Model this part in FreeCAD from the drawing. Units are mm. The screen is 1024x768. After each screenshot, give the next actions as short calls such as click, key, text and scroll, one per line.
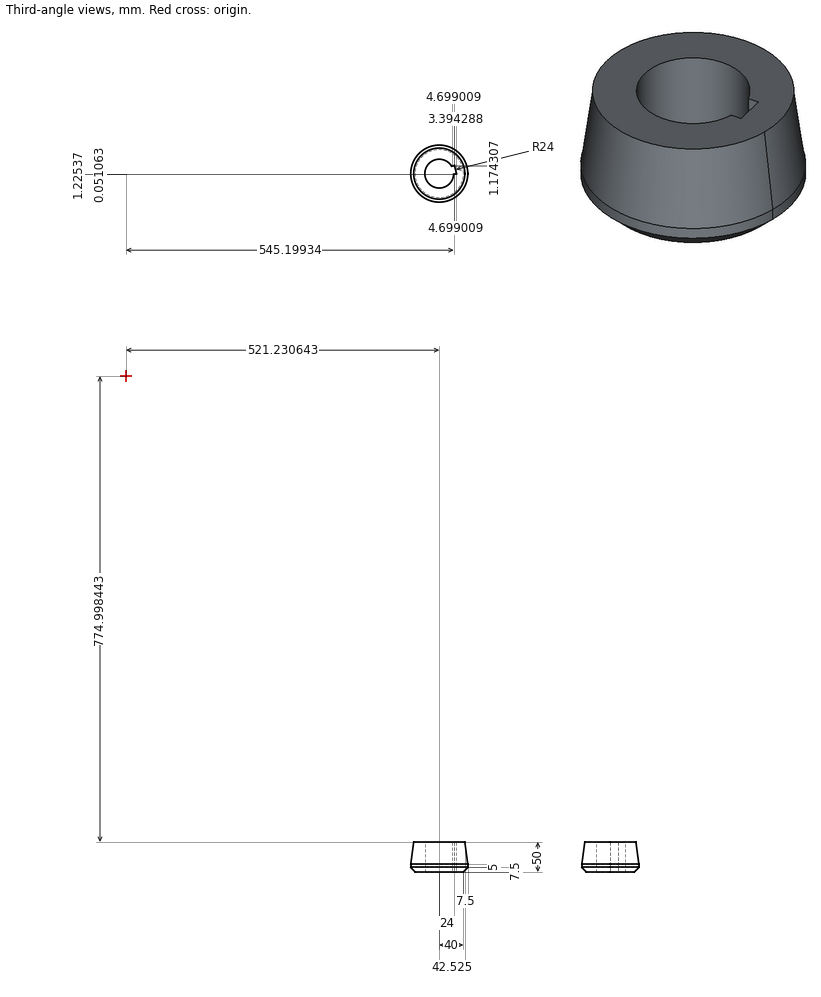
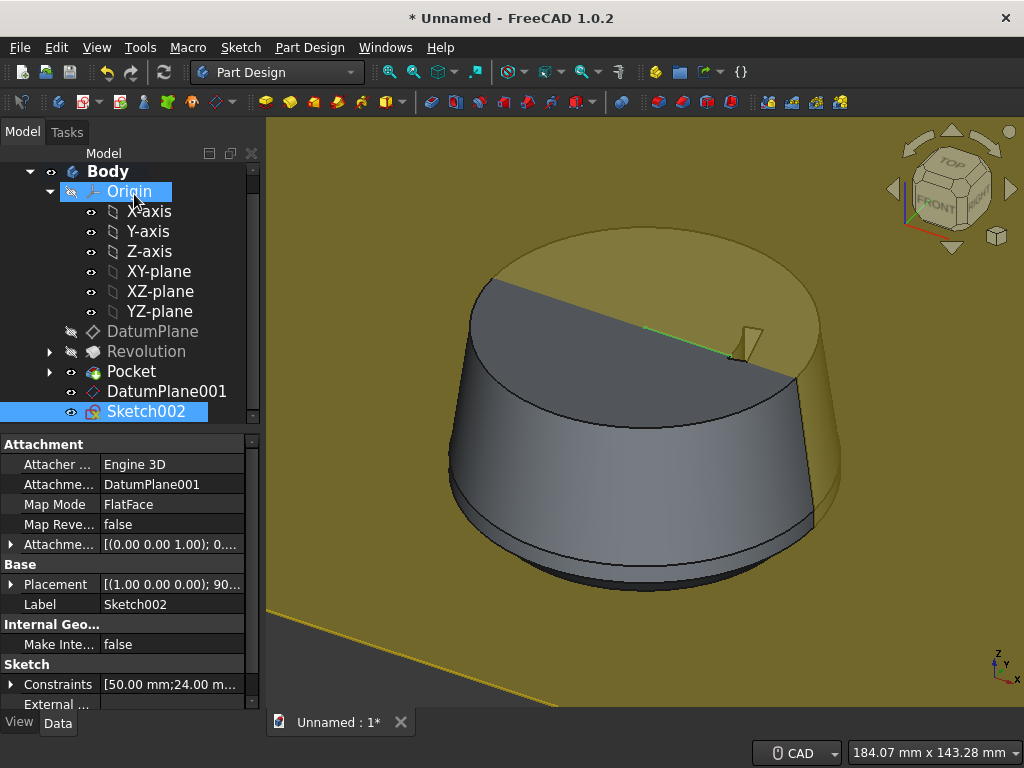
click(480, 102)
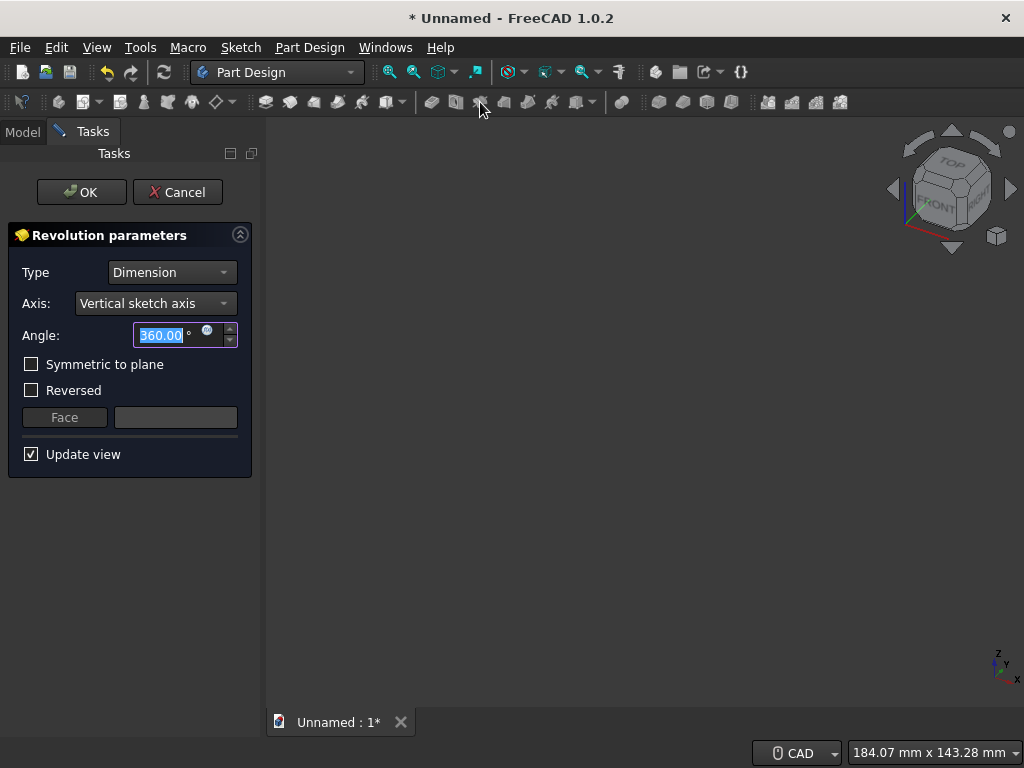
click(156, 304)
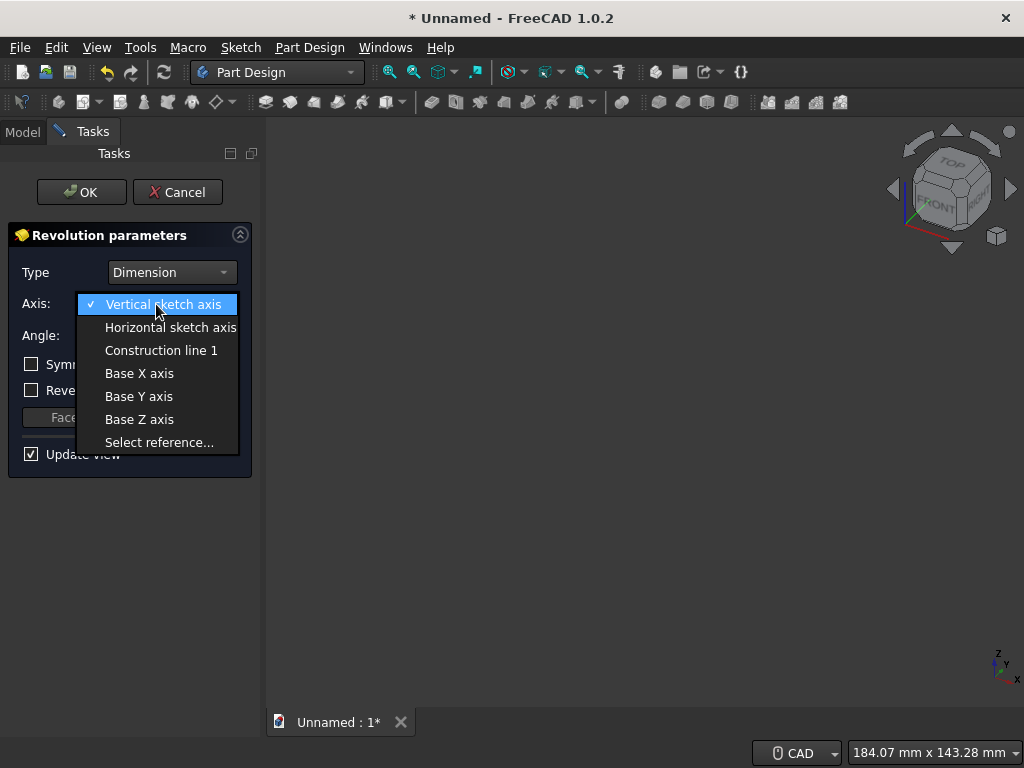
click(156, 350)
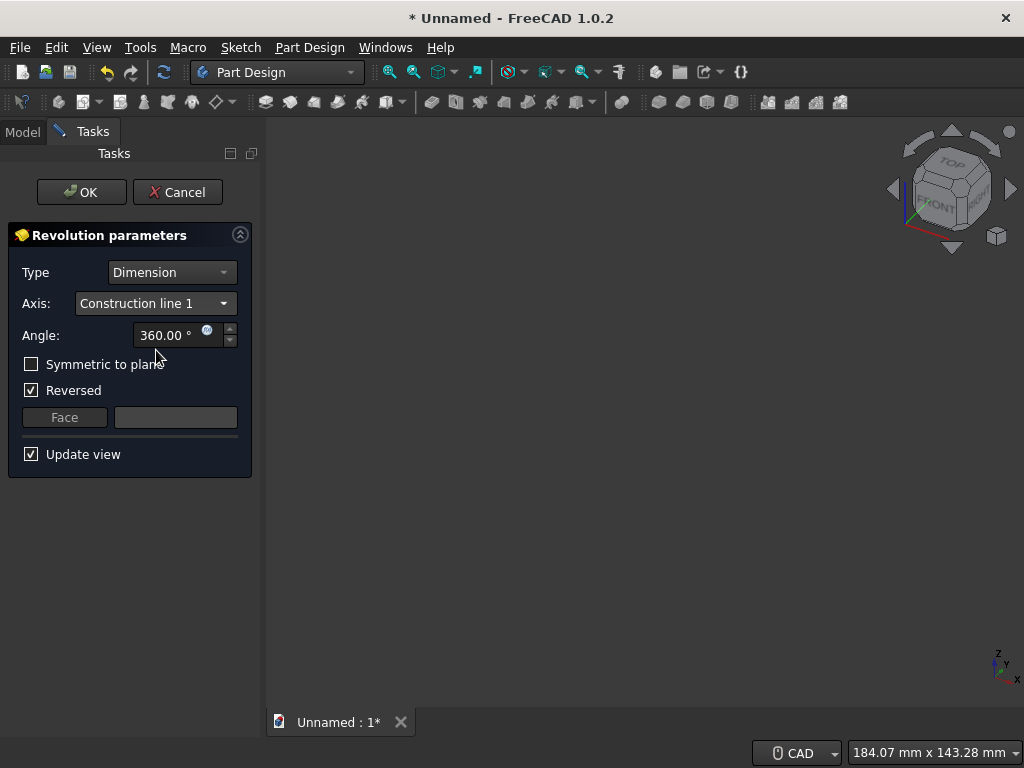
click(82, 192)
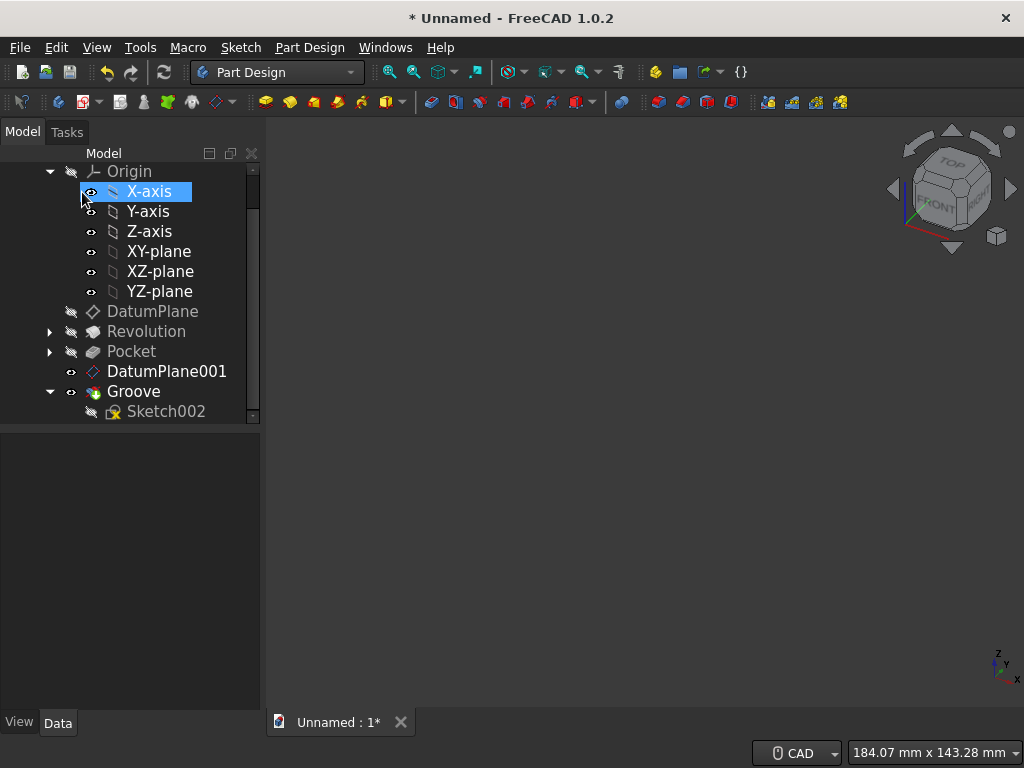
click(116, 372)
key(space)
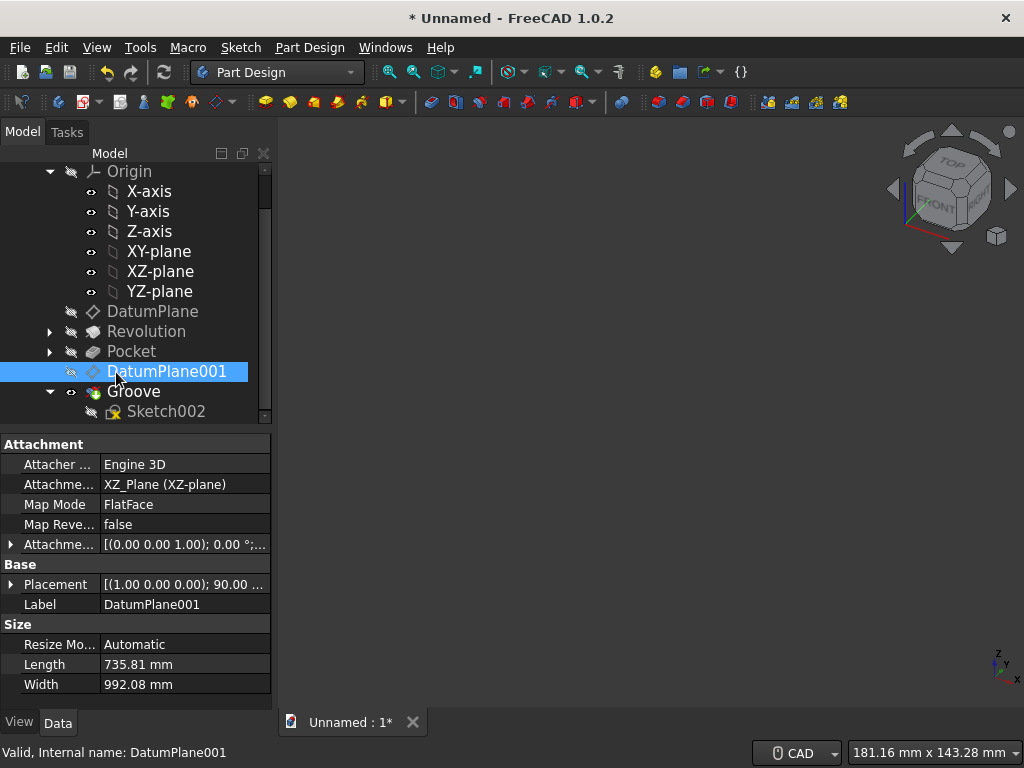
key(0)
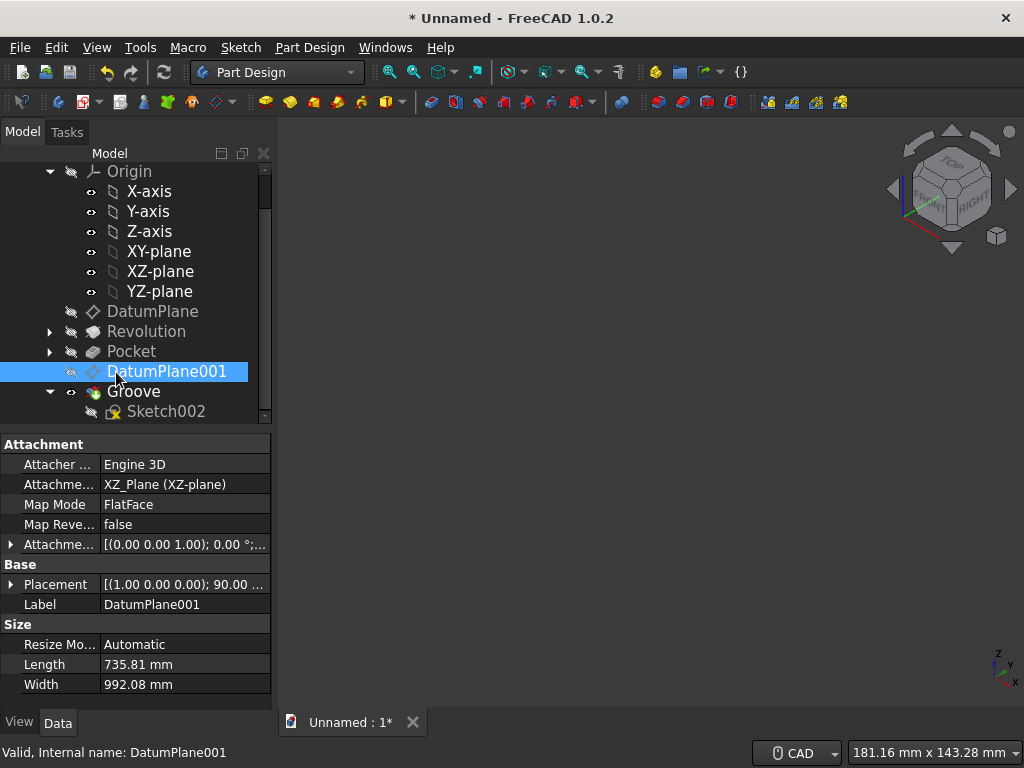
click(390, 72)